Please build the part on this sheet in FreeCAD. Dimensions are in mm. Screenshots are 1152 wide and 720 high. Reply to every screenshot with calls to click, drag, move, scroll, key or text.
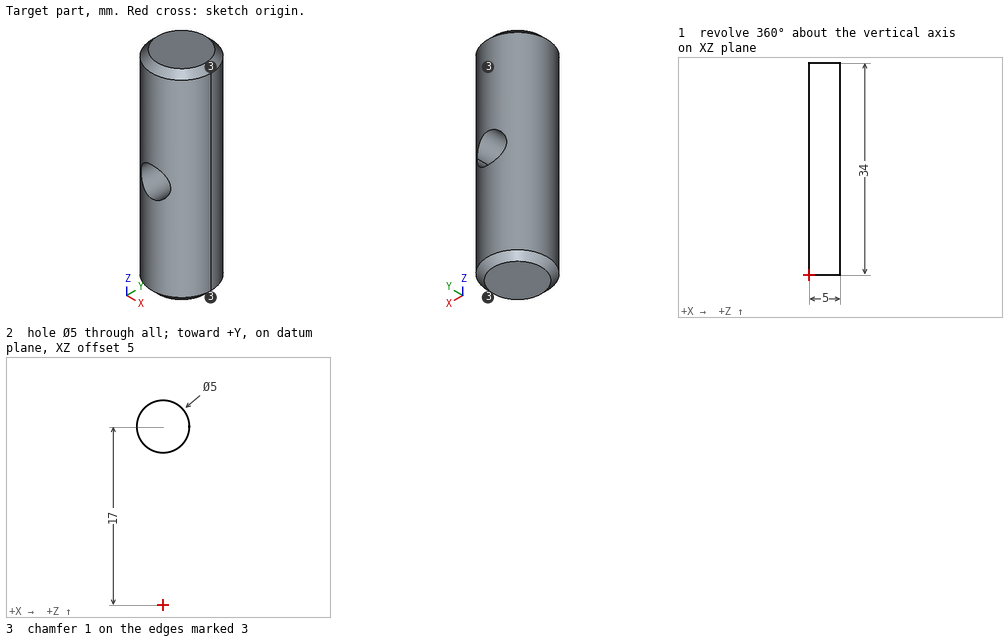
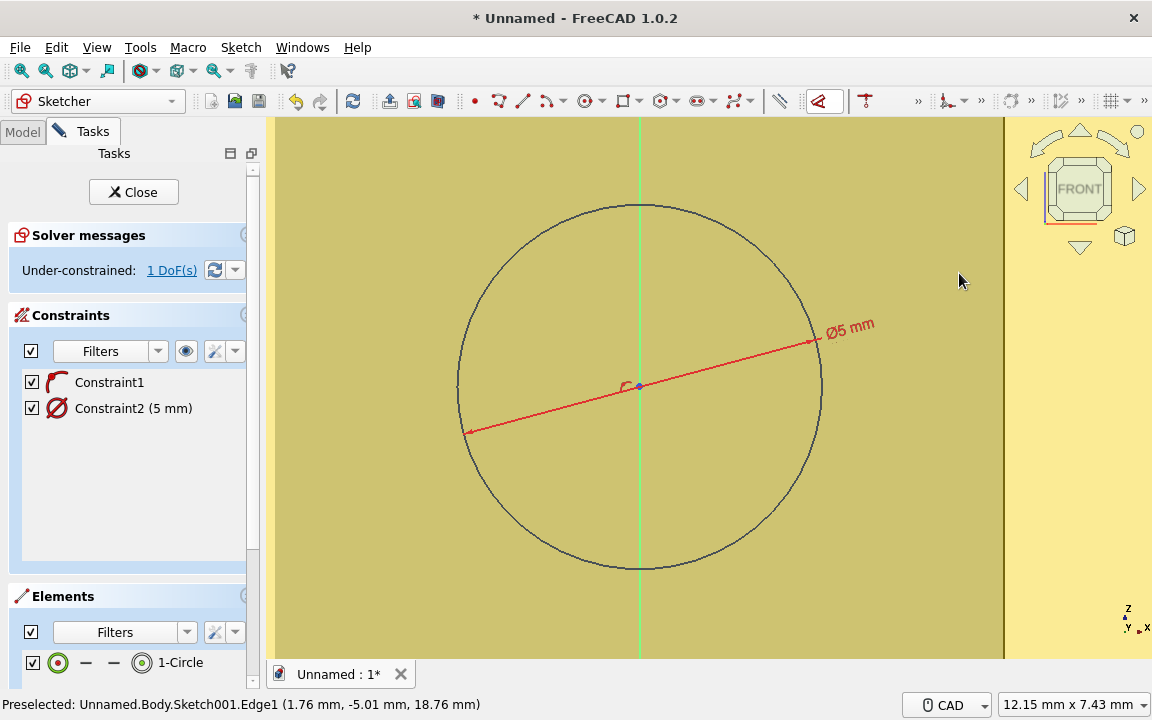
click(640, 387)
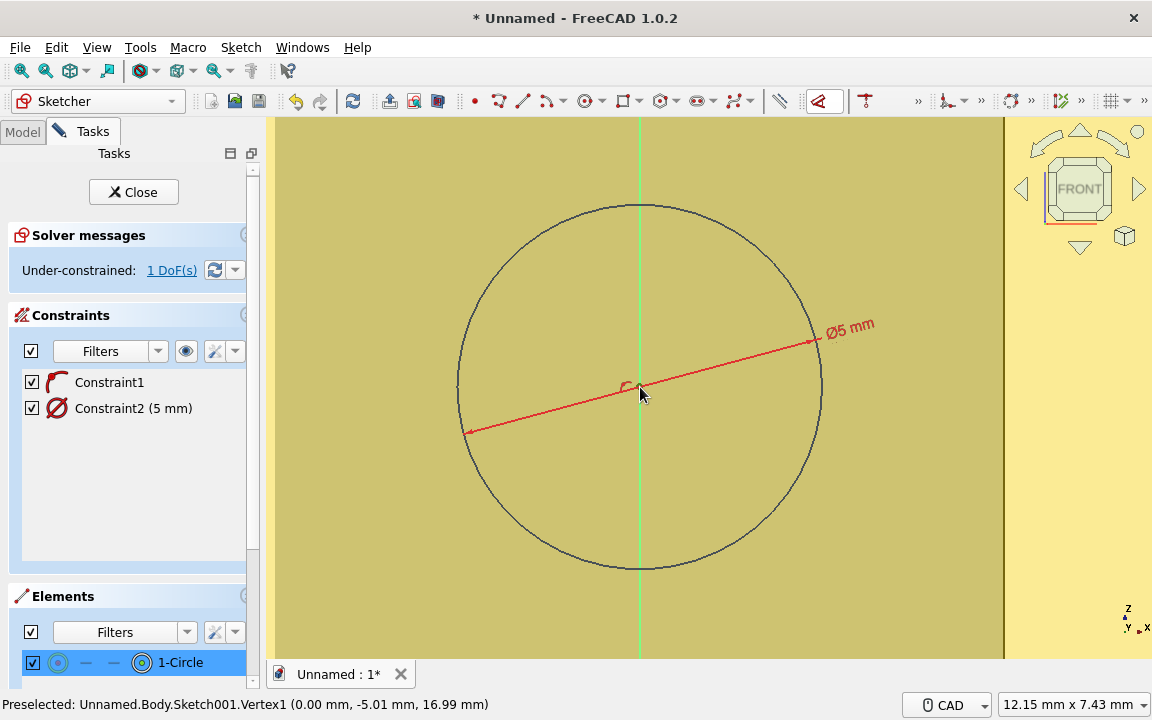
click(838, 102)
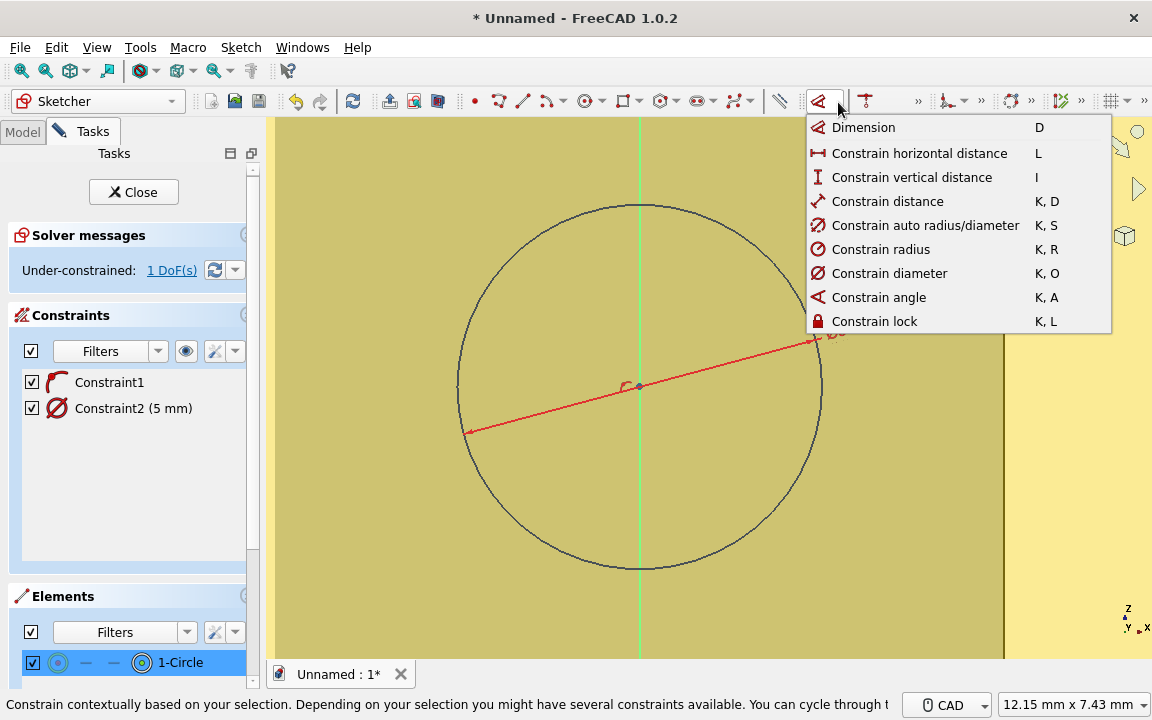
click(959, 177)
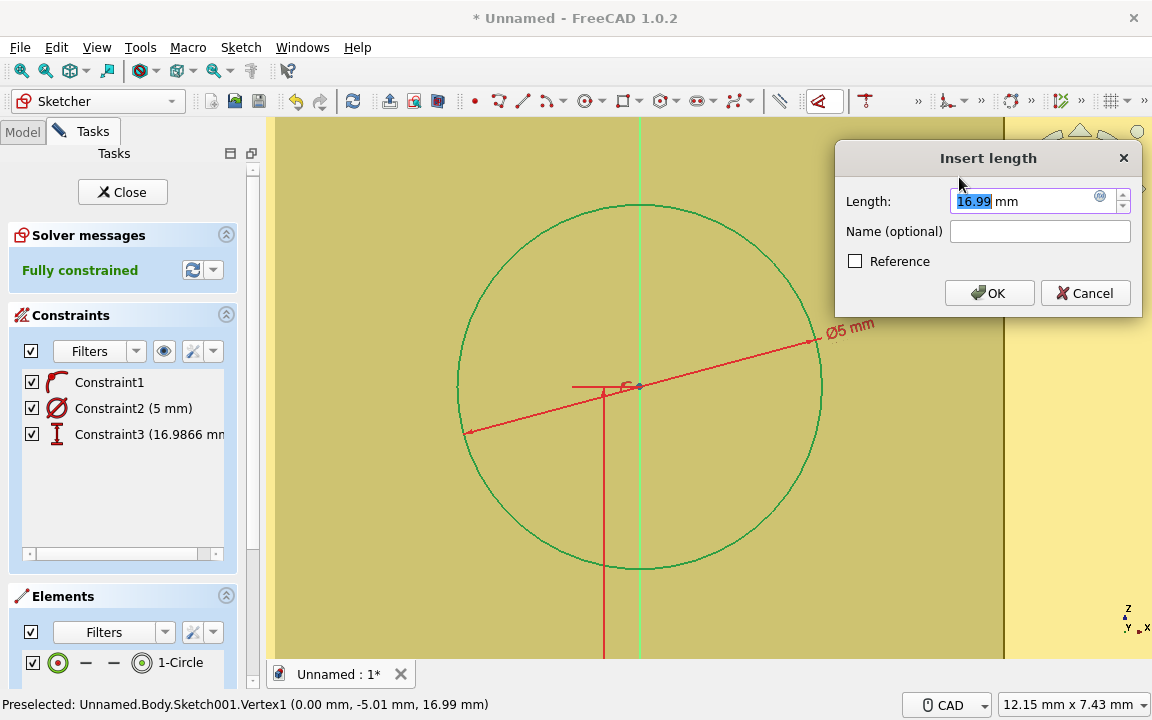
text(17)
key(Return)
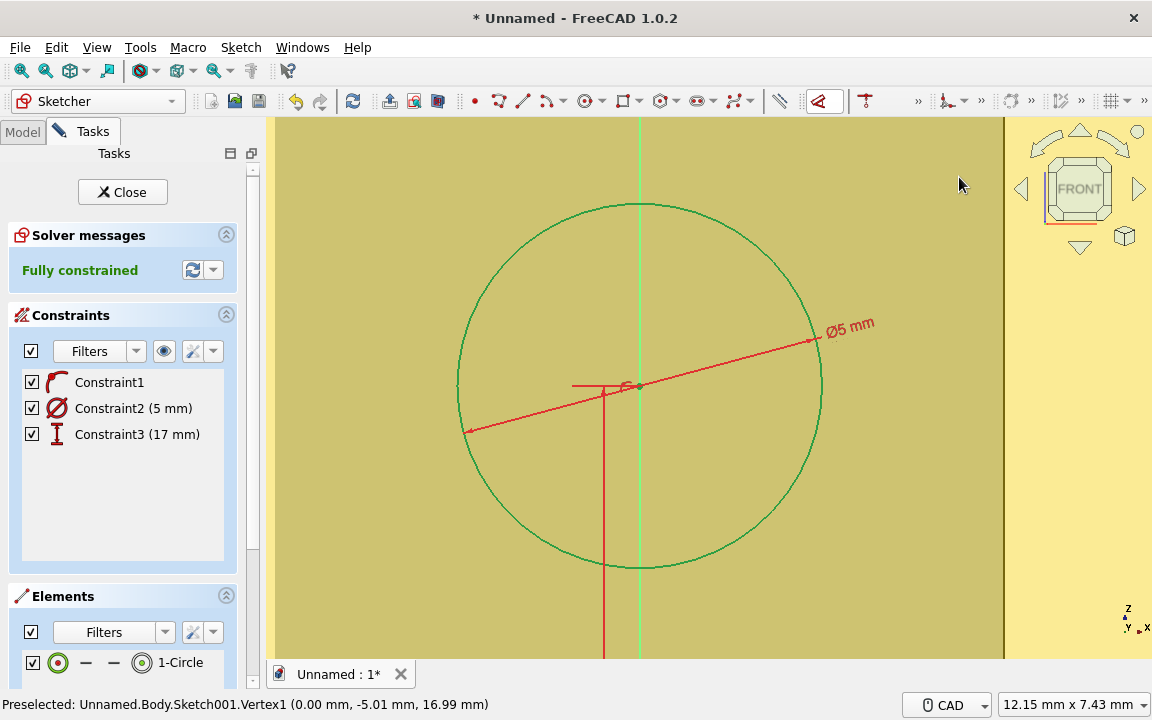
click(123, 192)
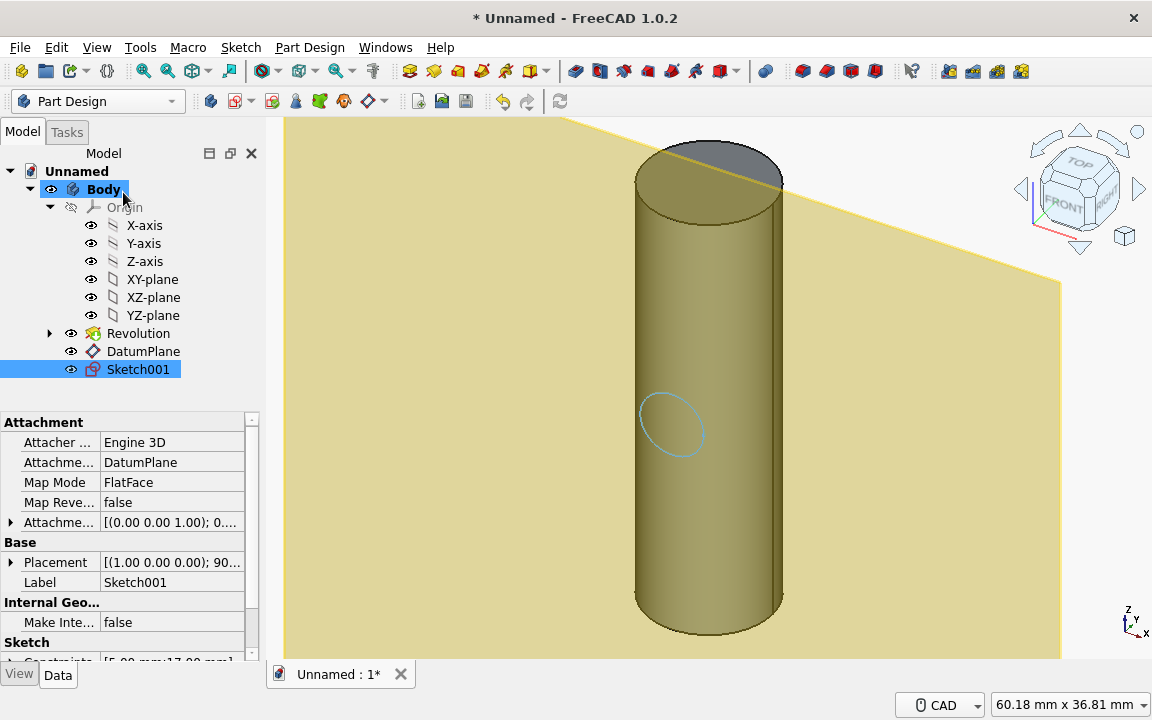
click(600, 72)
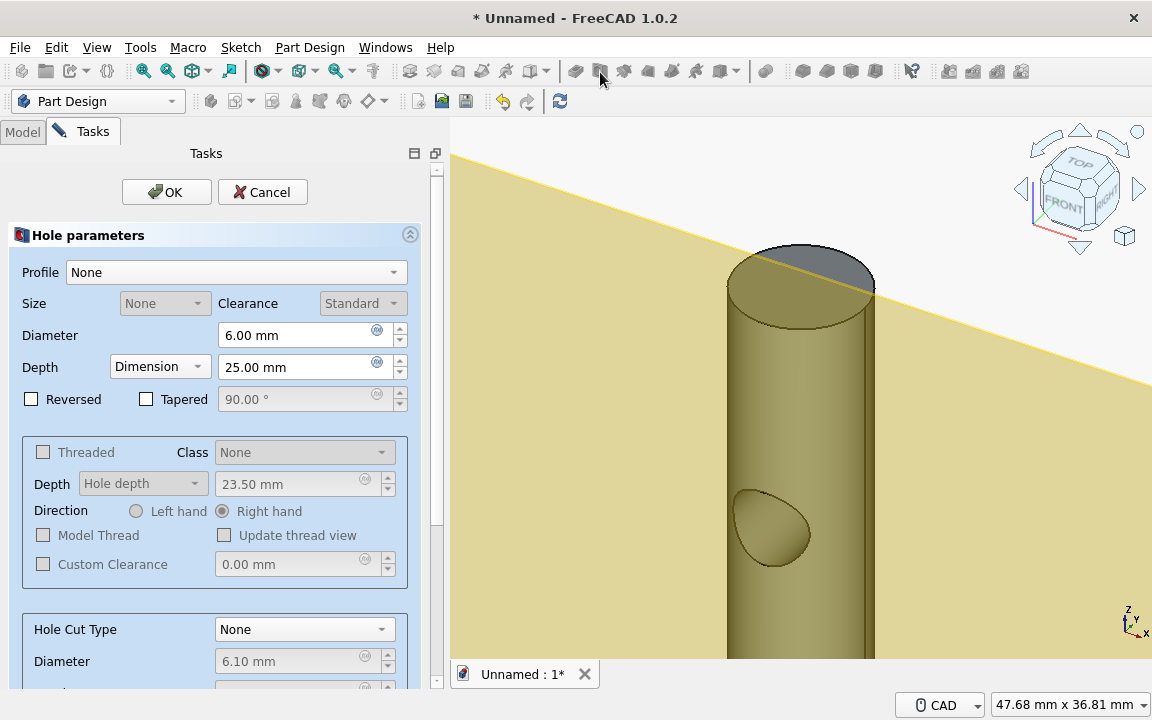
triple_click(305, 335)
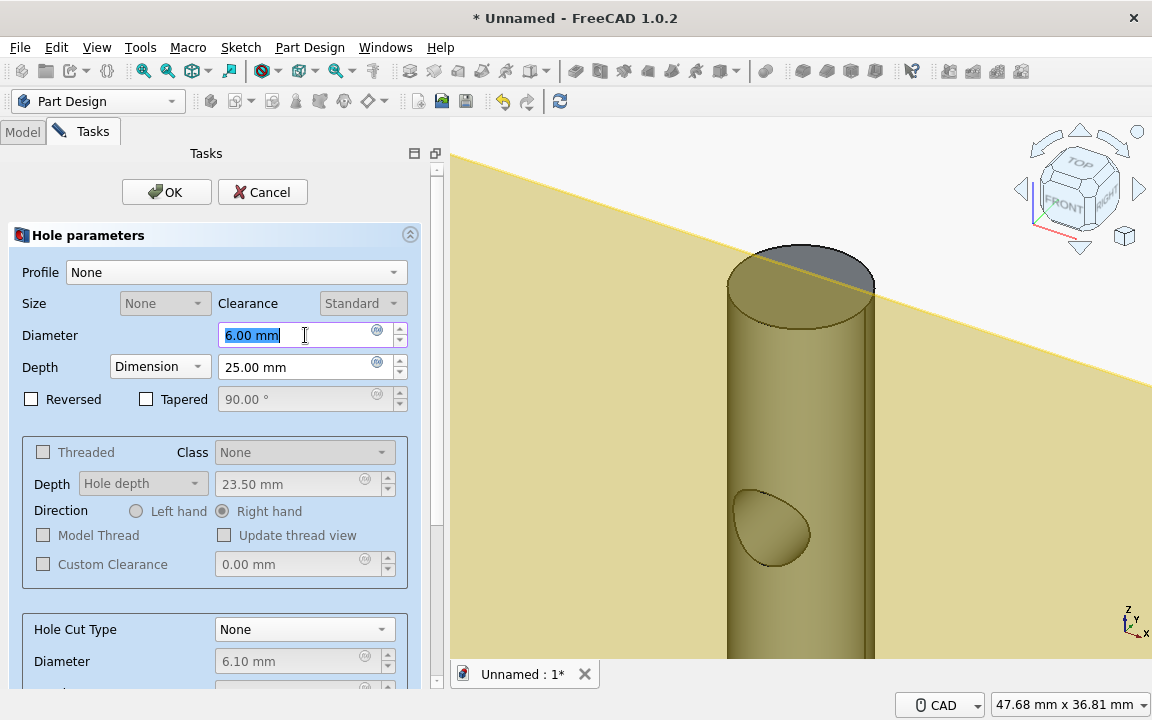
text(5)
key(Tab)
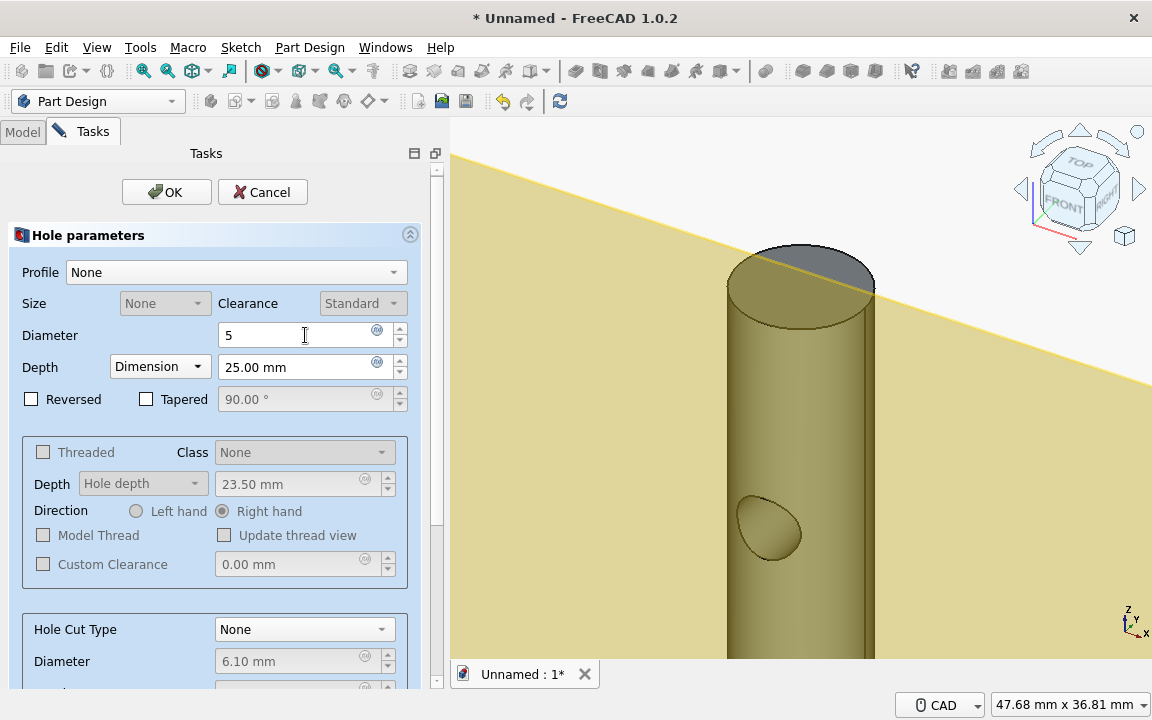
click(161, 366)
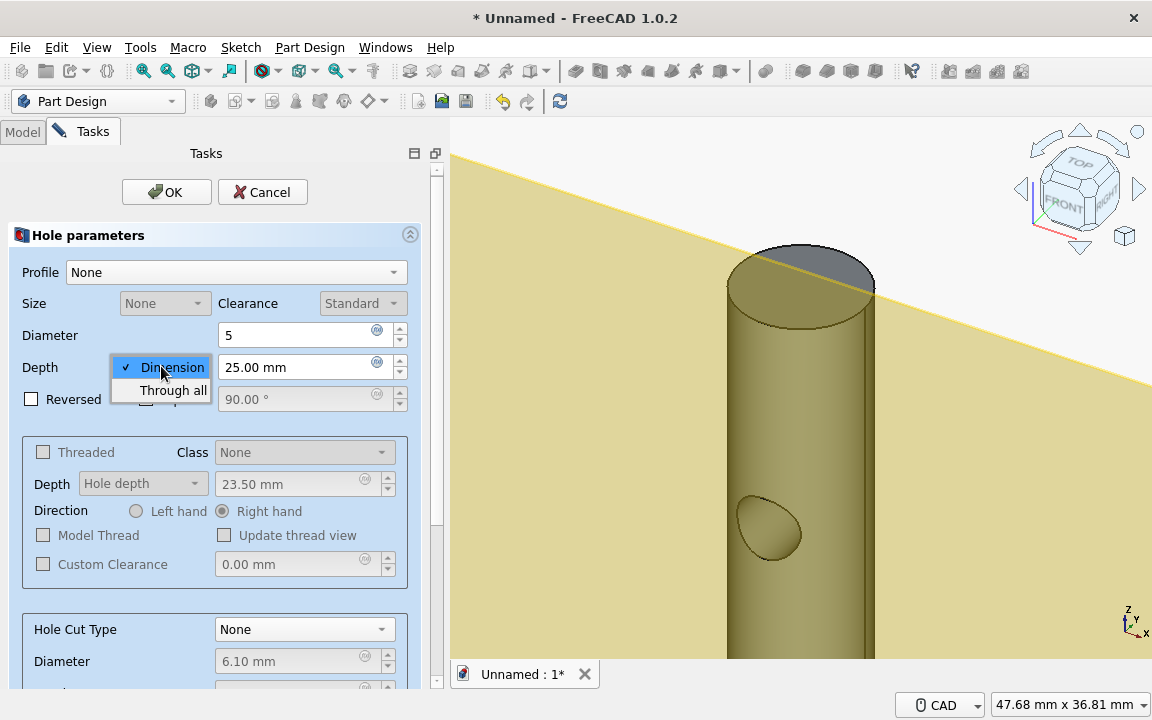
click(160, 390)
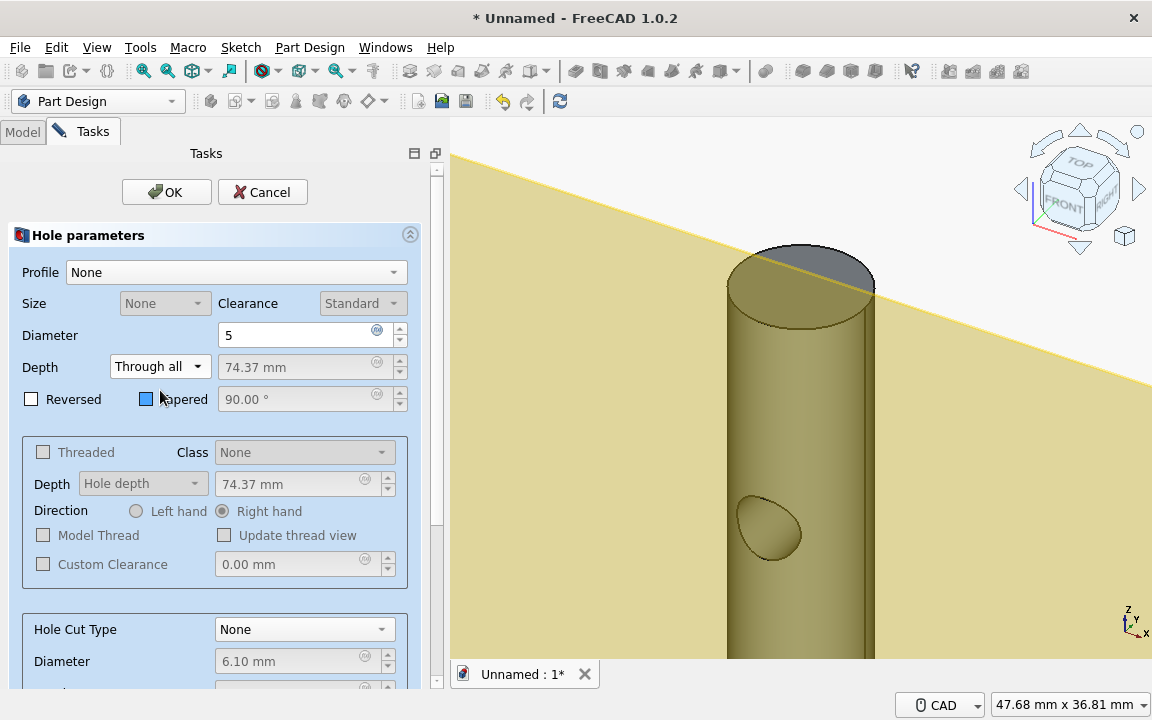
click(167, 192)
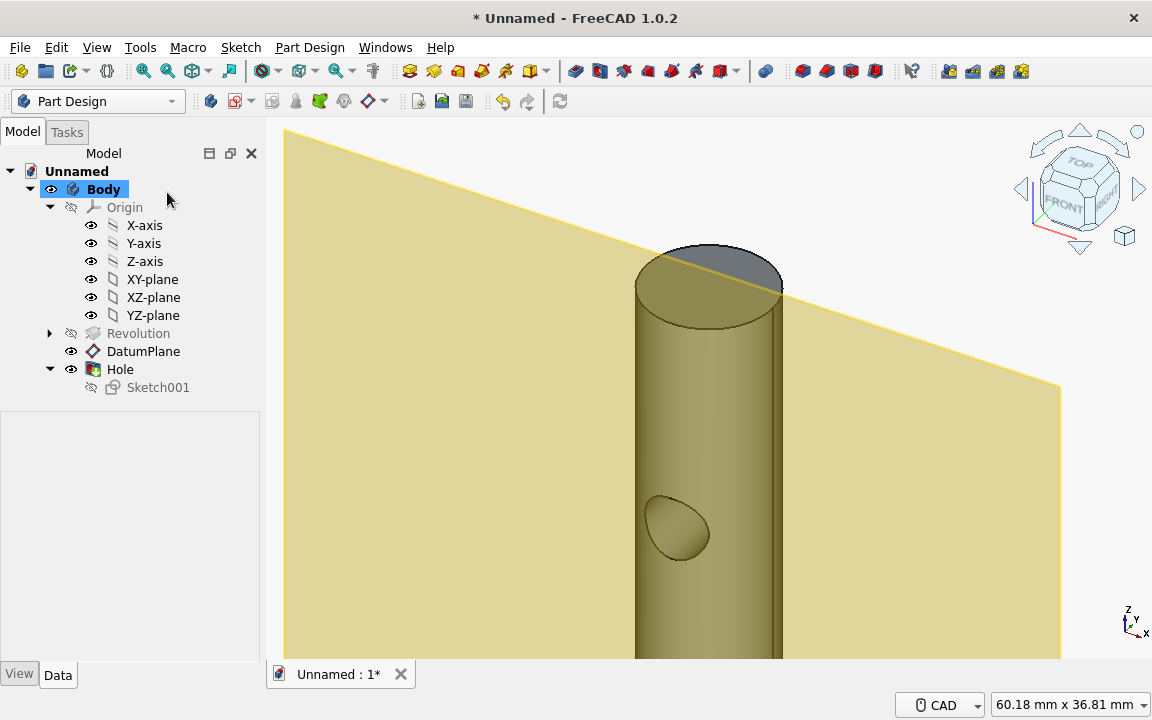
click(116, 351)
key(space)